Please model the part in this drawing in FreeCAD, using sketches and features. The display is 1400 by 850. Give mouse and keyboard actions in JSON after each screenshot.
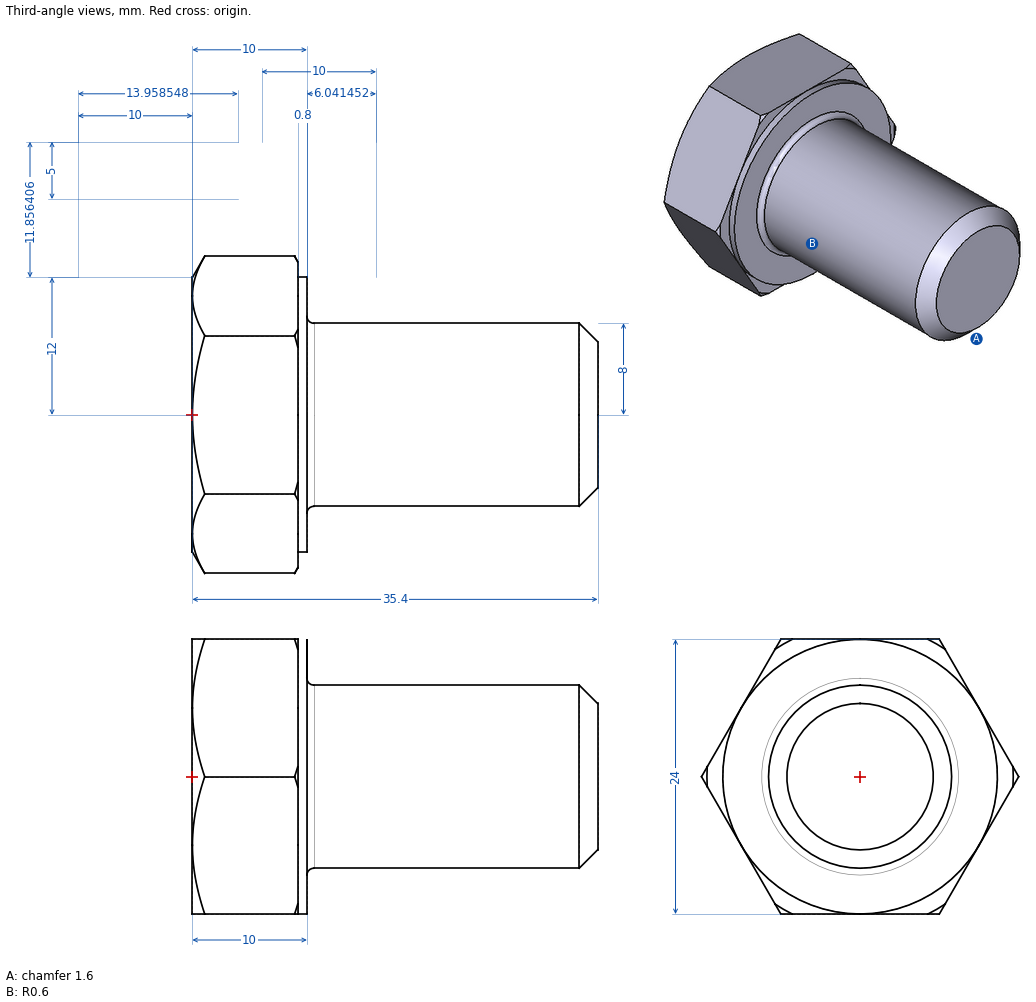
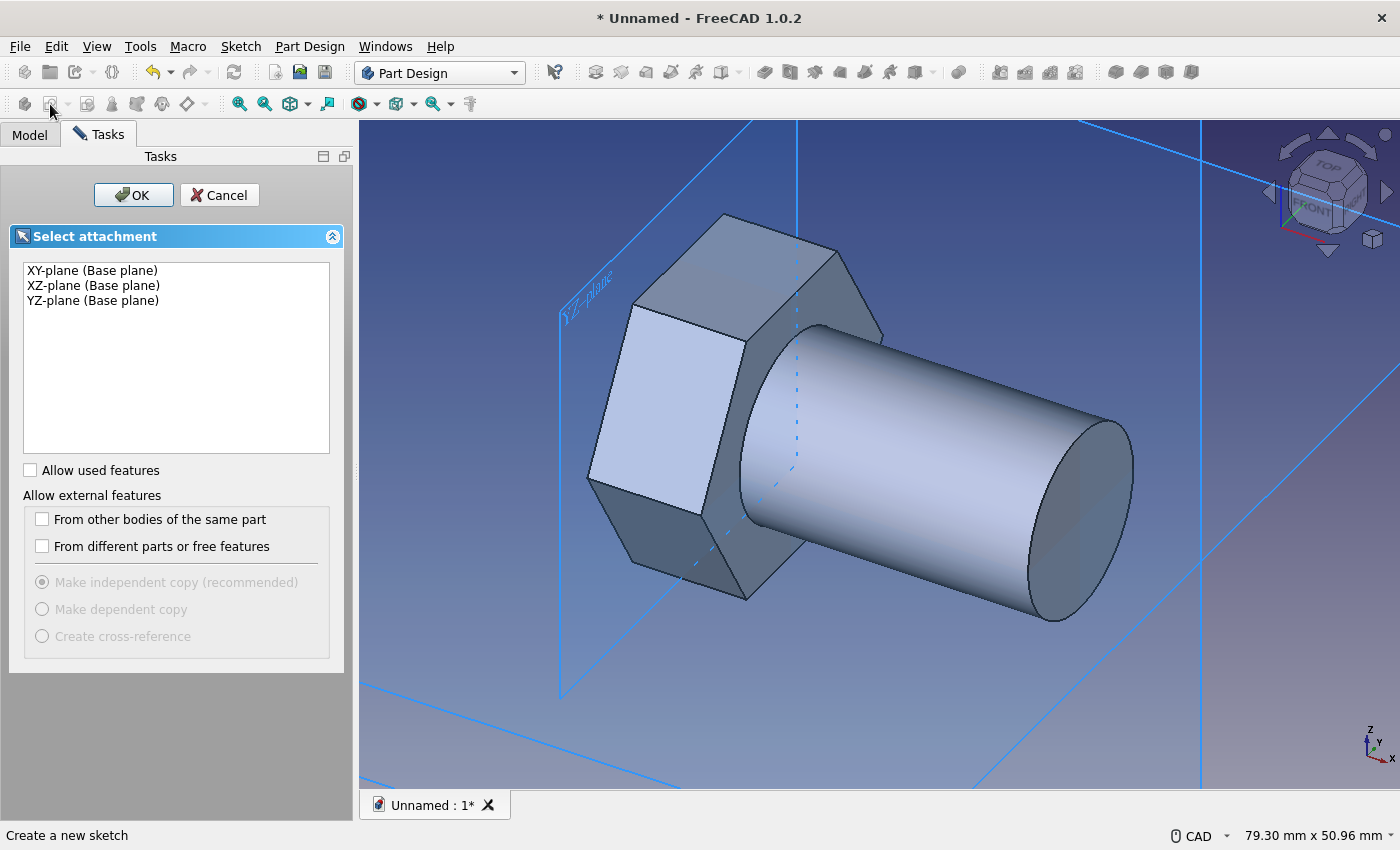
{"action": "left_click", "coordinate": [84, 270]}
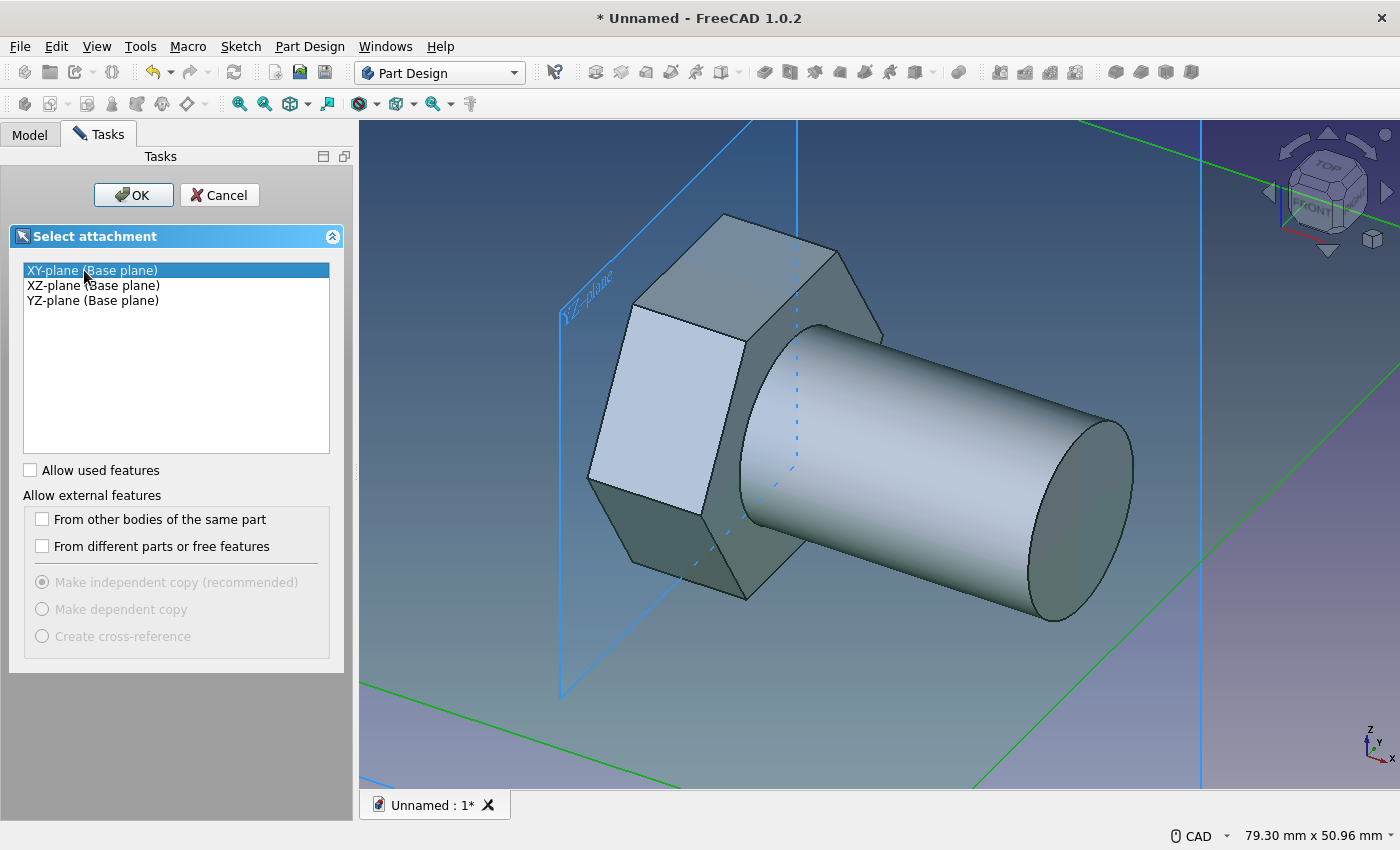
{"action": "left_click", "coordinate": [134, 195]}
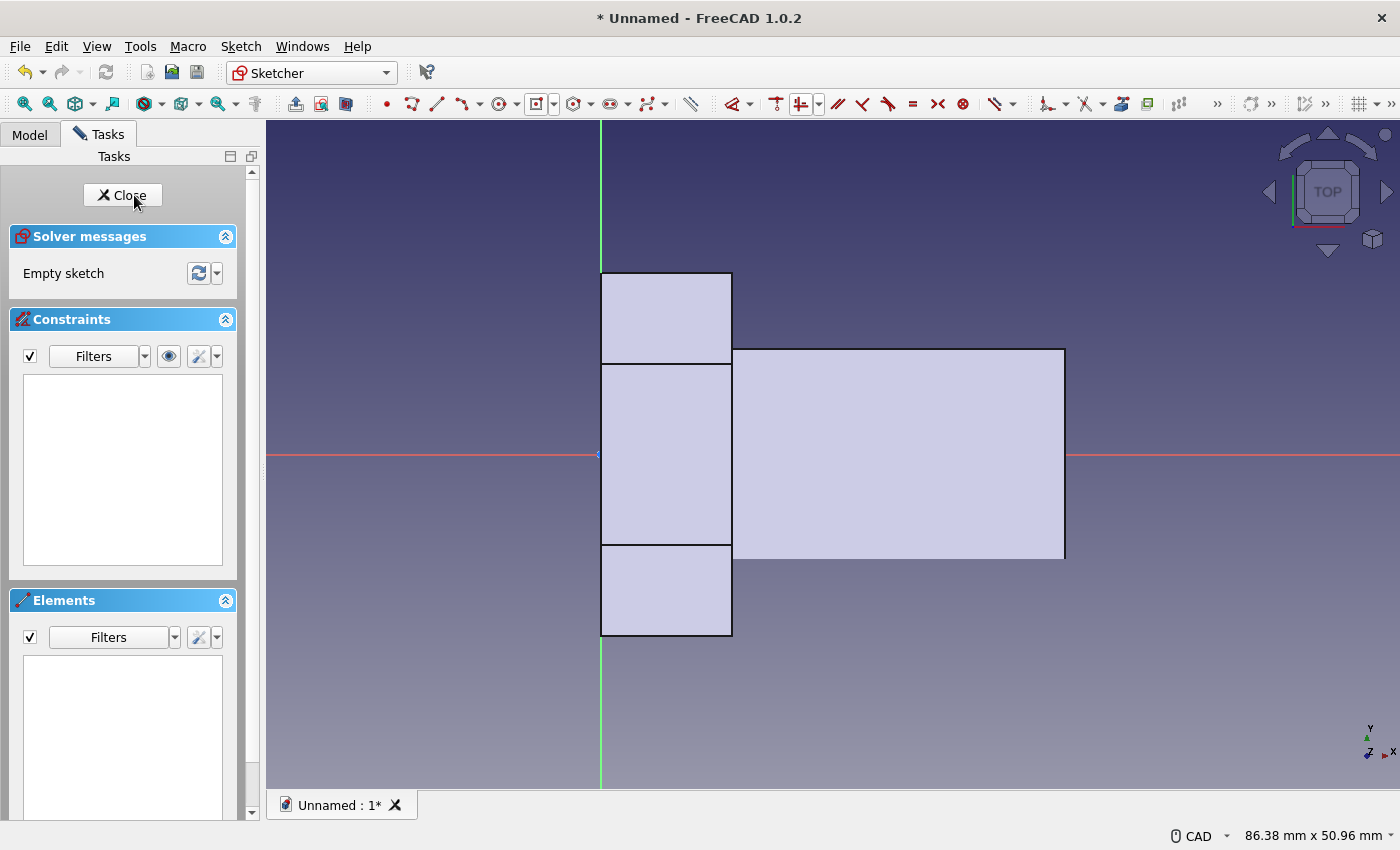
{"action": "key", "text": "q s"}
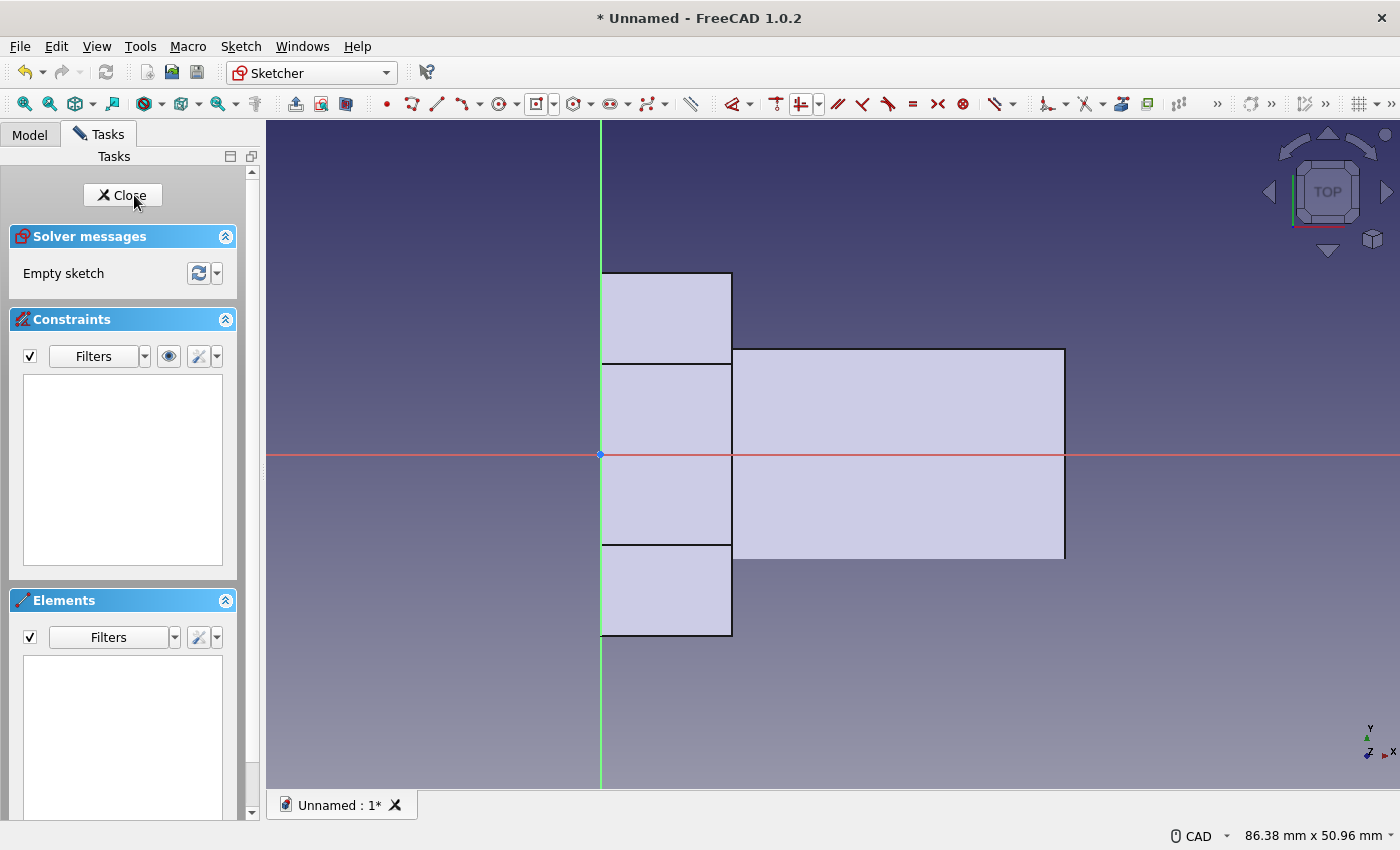
{"action": "scroll", "coordinate": [1235, 761], "scroll_direction": "down", "scroll_amount": 1}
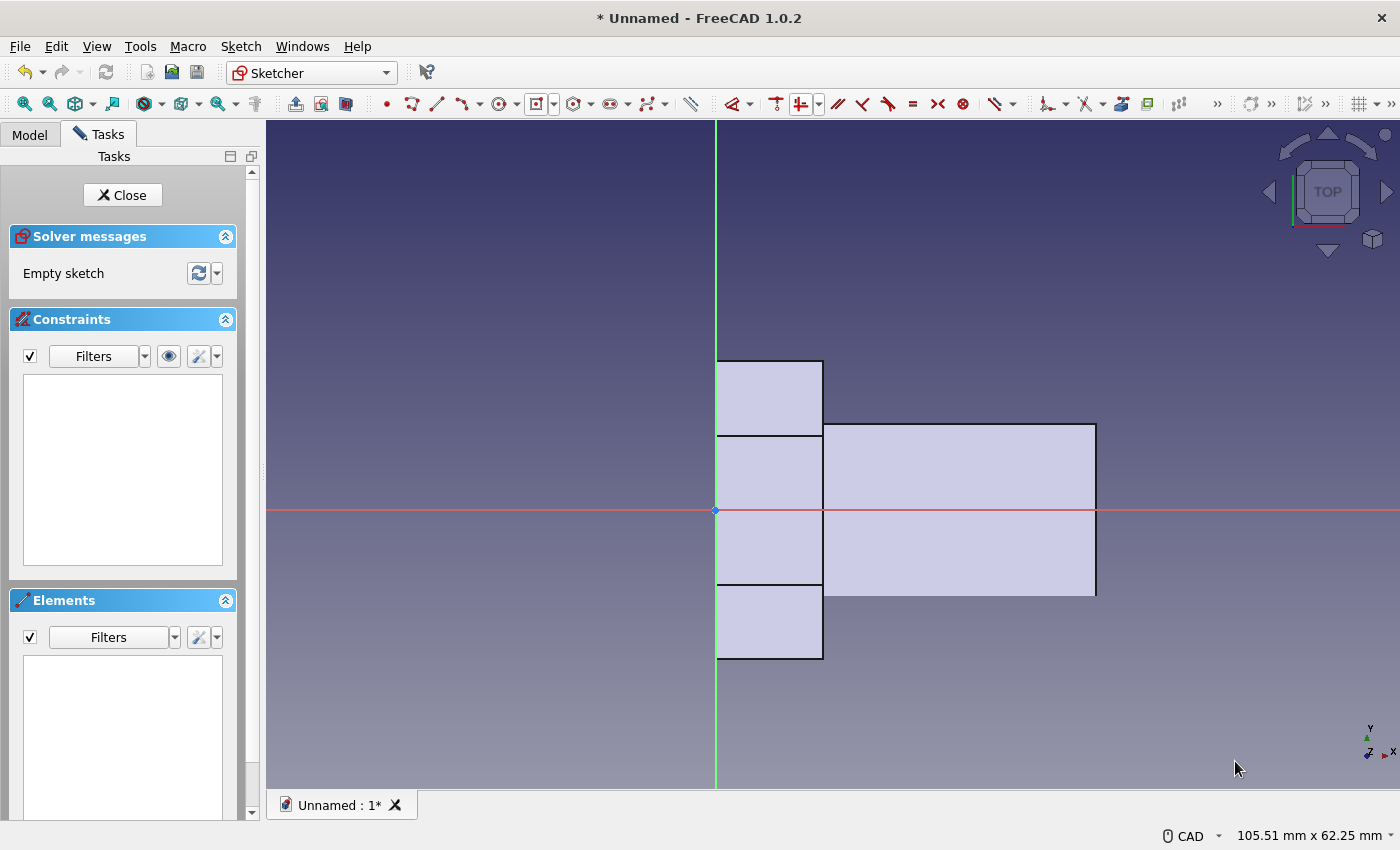
{"action": "scroll", "coordinate": [585, 294], "scroll_direction": "up", "scroll_amount": 3}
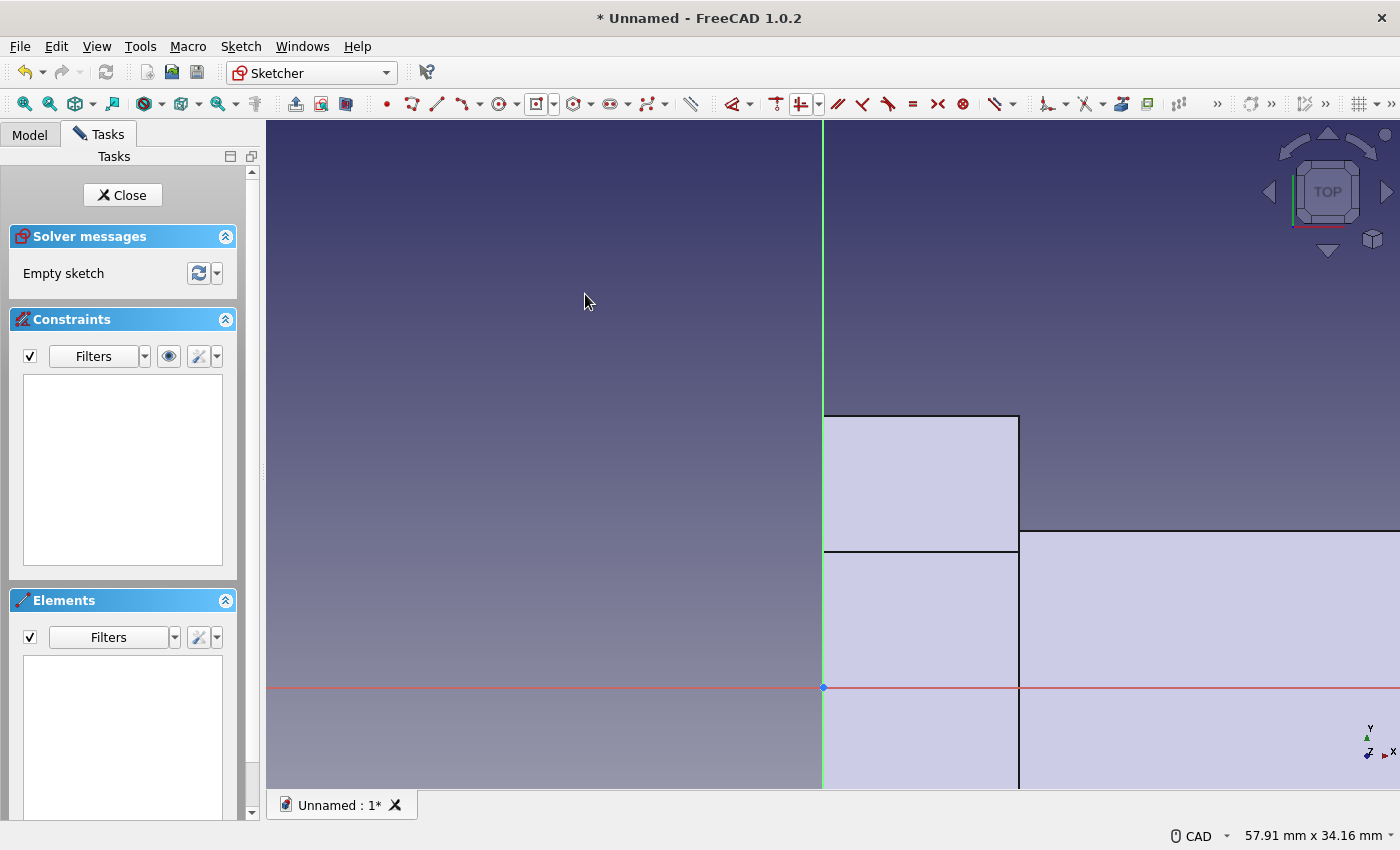
{"action": "key", "text": "g m"}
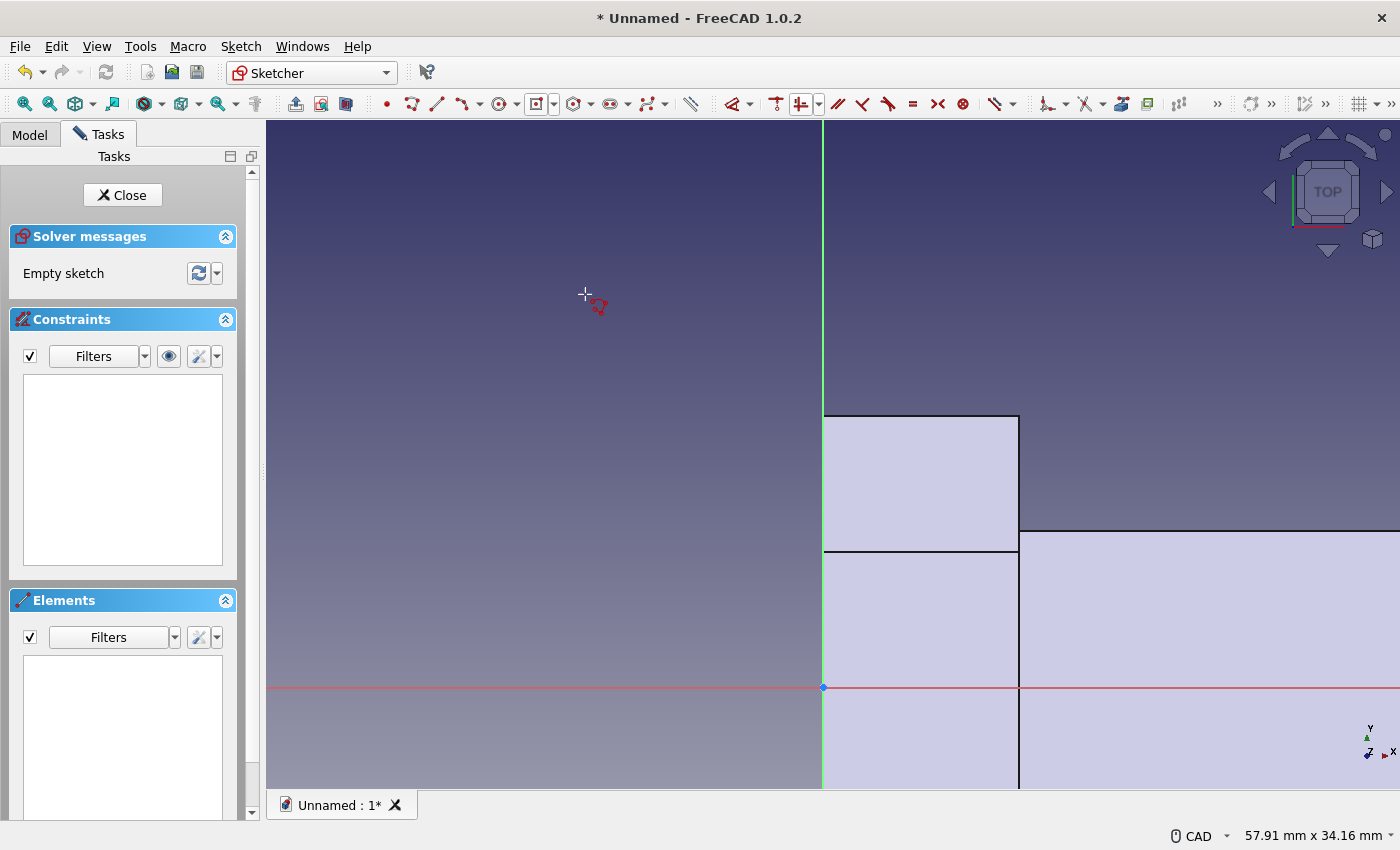
{"action": "left_click", "coordinate": [823, 453]}
{"action": "left_click", "coordinate": [901, 319]}
{"action": "left_click", "coordinate": [901, 221]}
{"action": "left_click", "coordinate": [627, 221]}
{"action": "left_click", "coordinate": [627, 453]}
{"action": "left_click", "coordinate": [823, 454]}
{"action": "key", "text": "Escape"}
{"action": "key", "text": "Escape"}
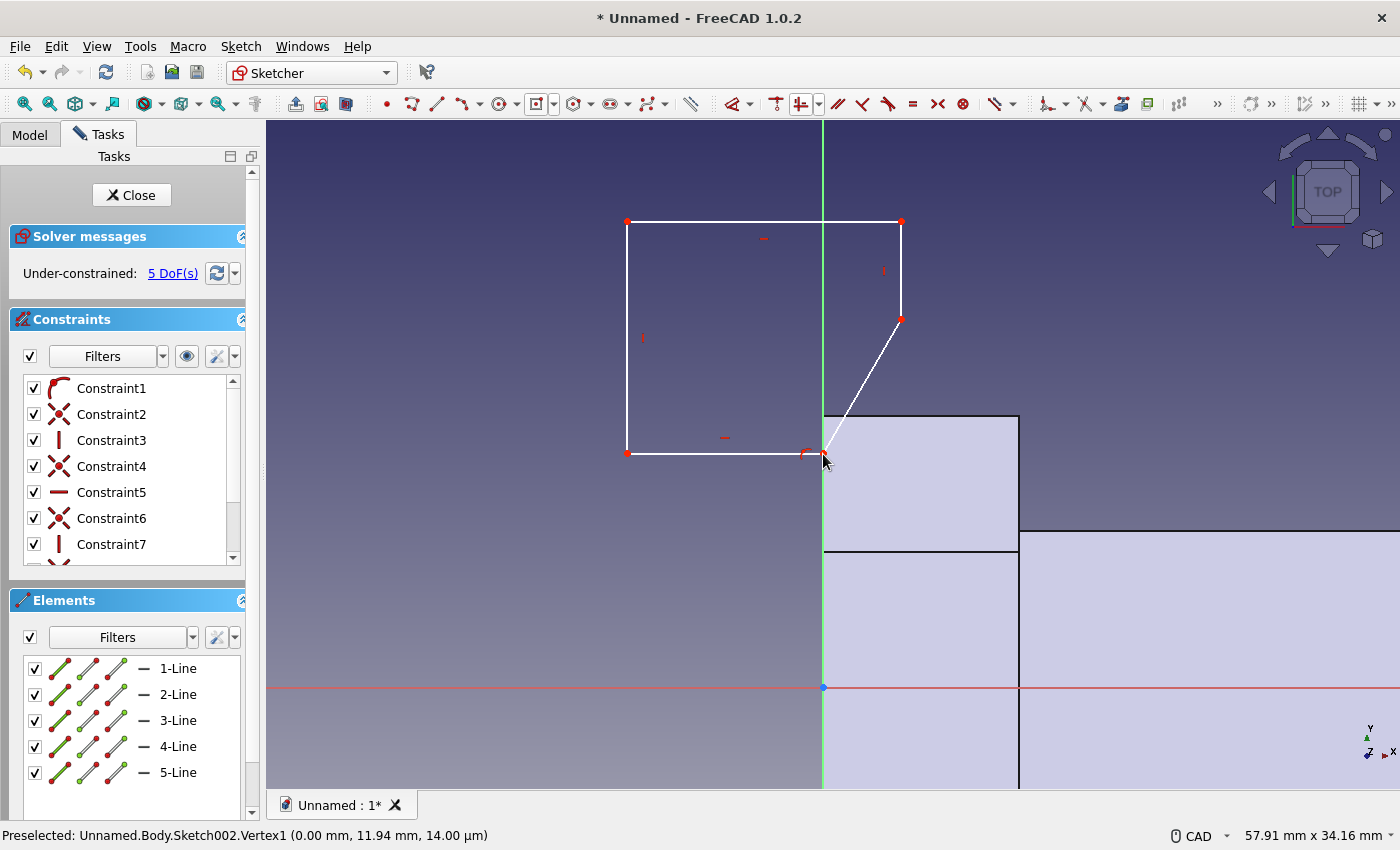
{"action": "key", "text": "d"}